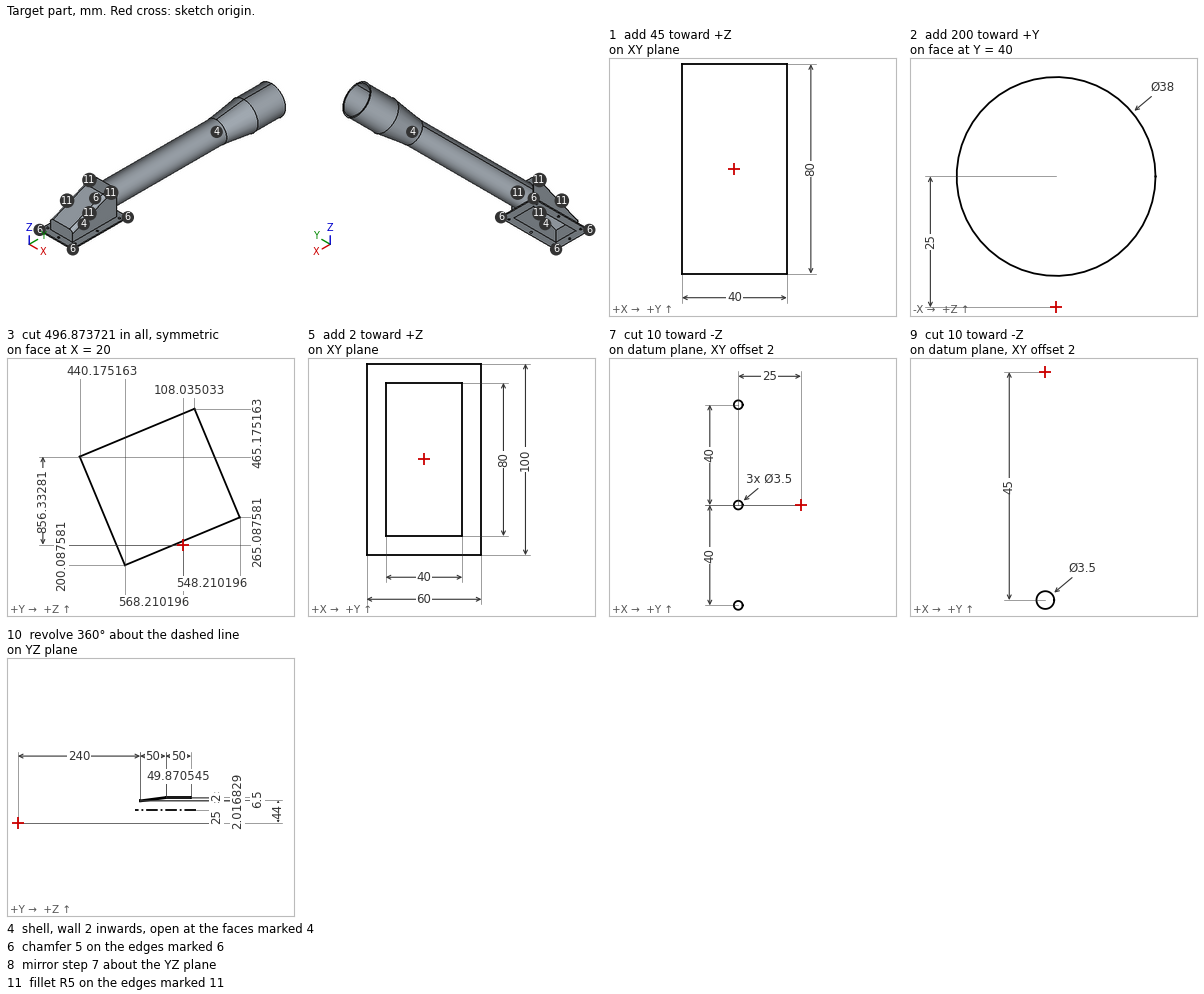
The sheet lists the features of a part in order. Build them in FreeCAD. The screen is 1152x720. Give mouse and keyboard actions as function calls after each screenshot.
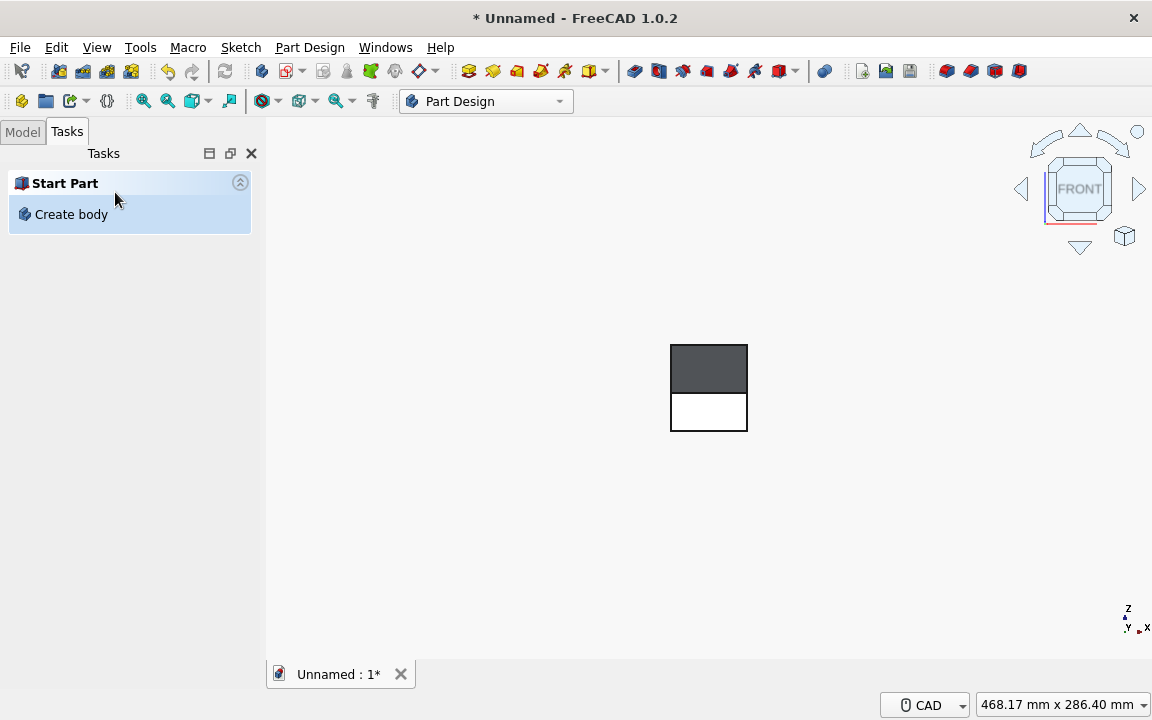
key(3)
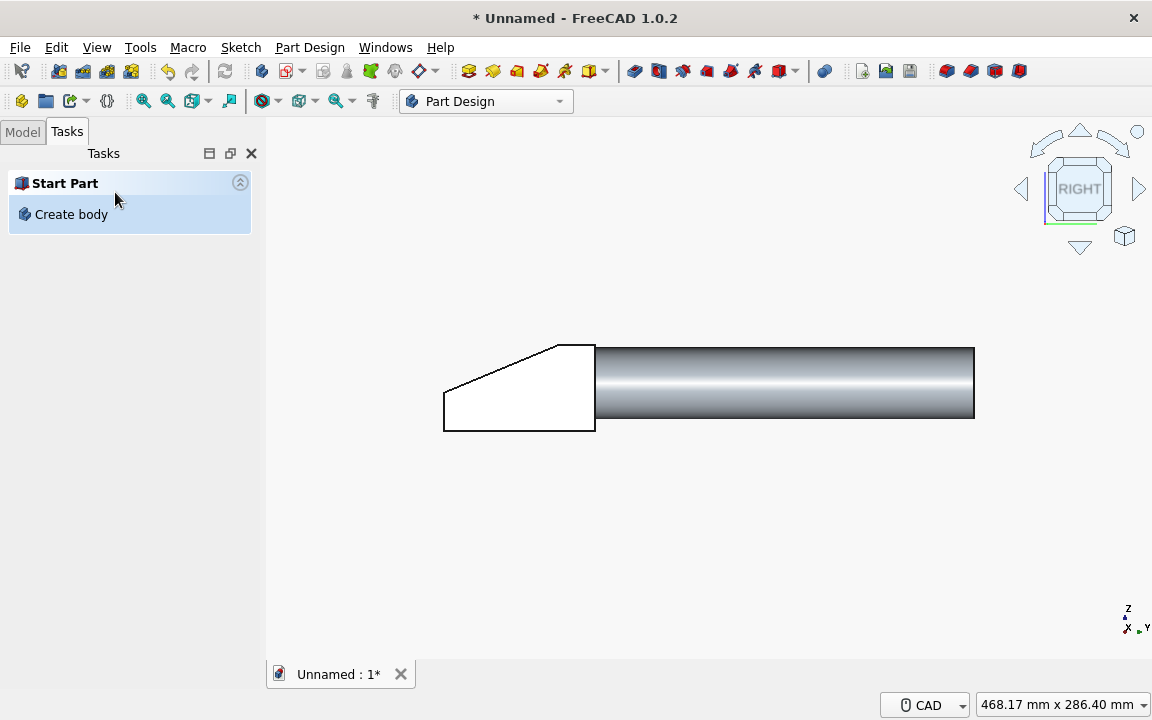
key(5)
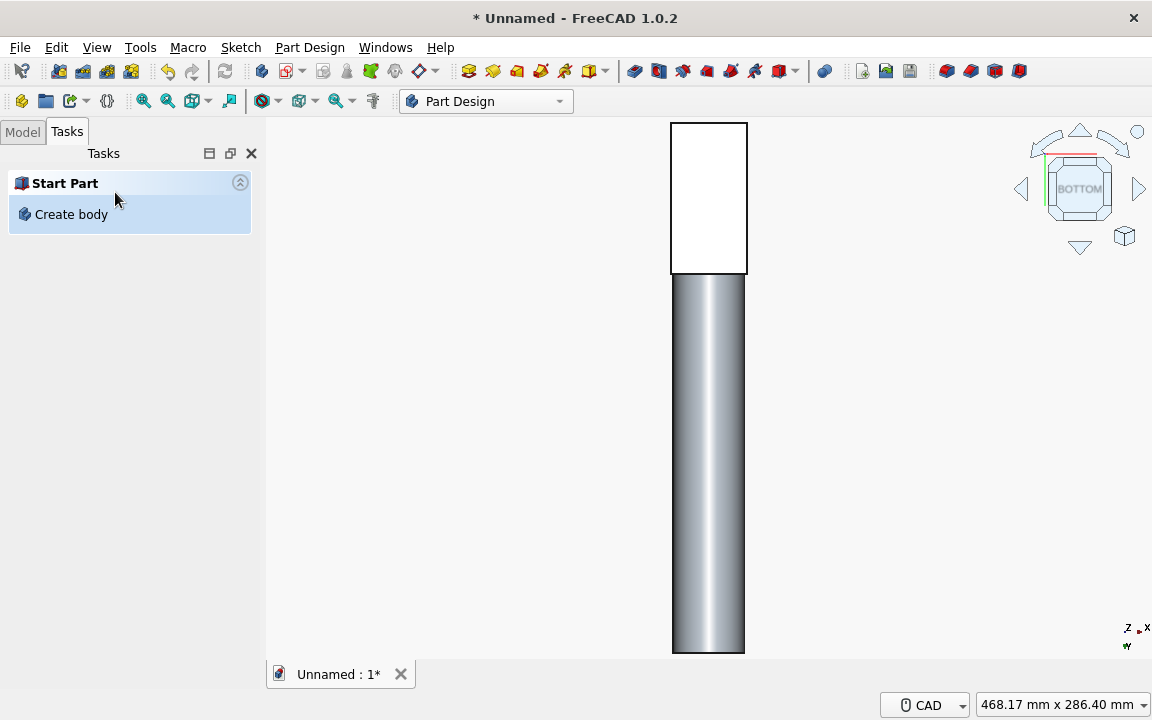
click(709, 219)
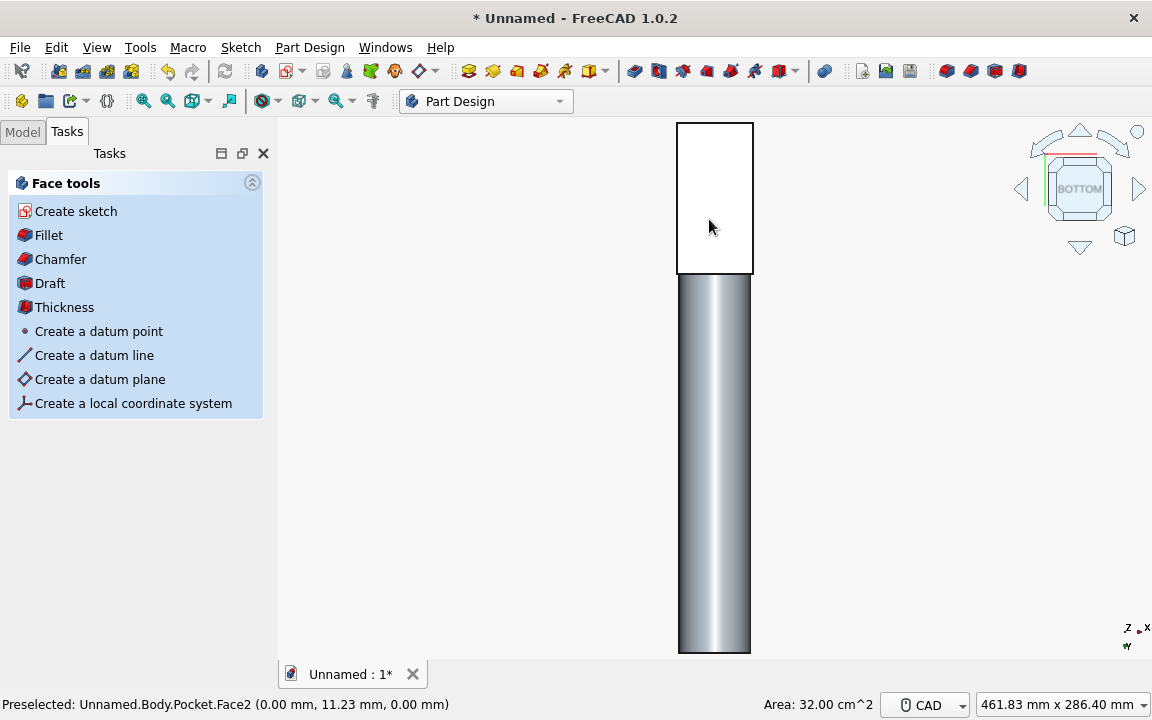
key(4)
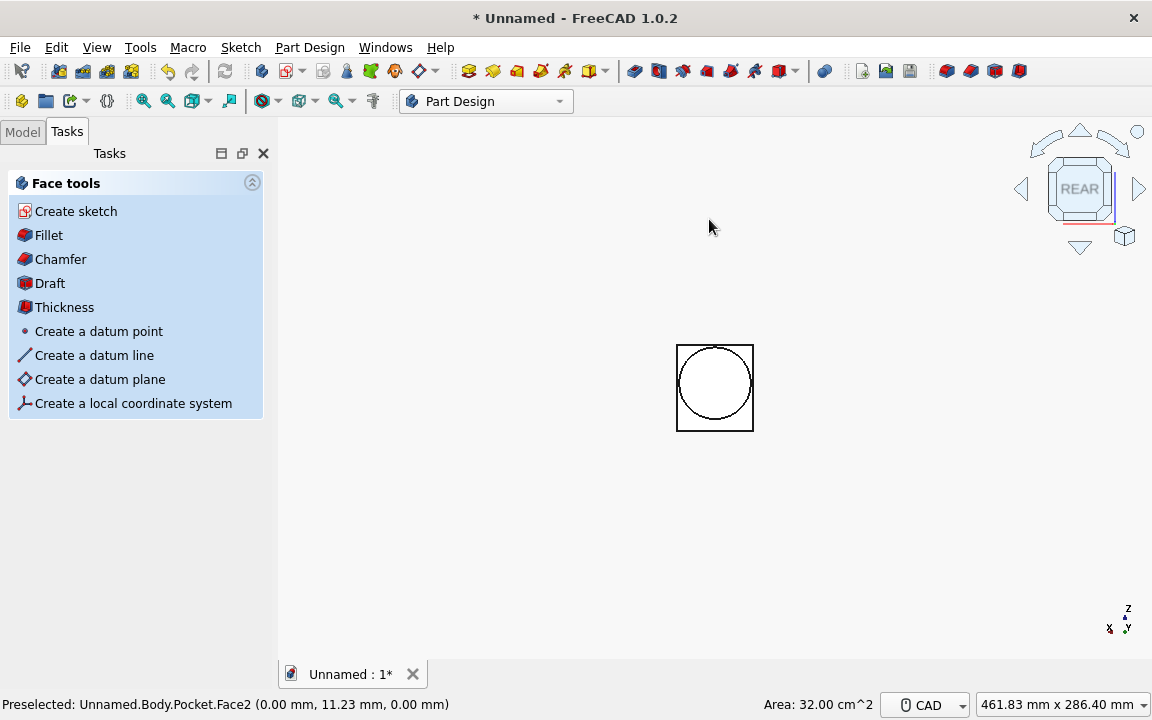
key(v)
key(f)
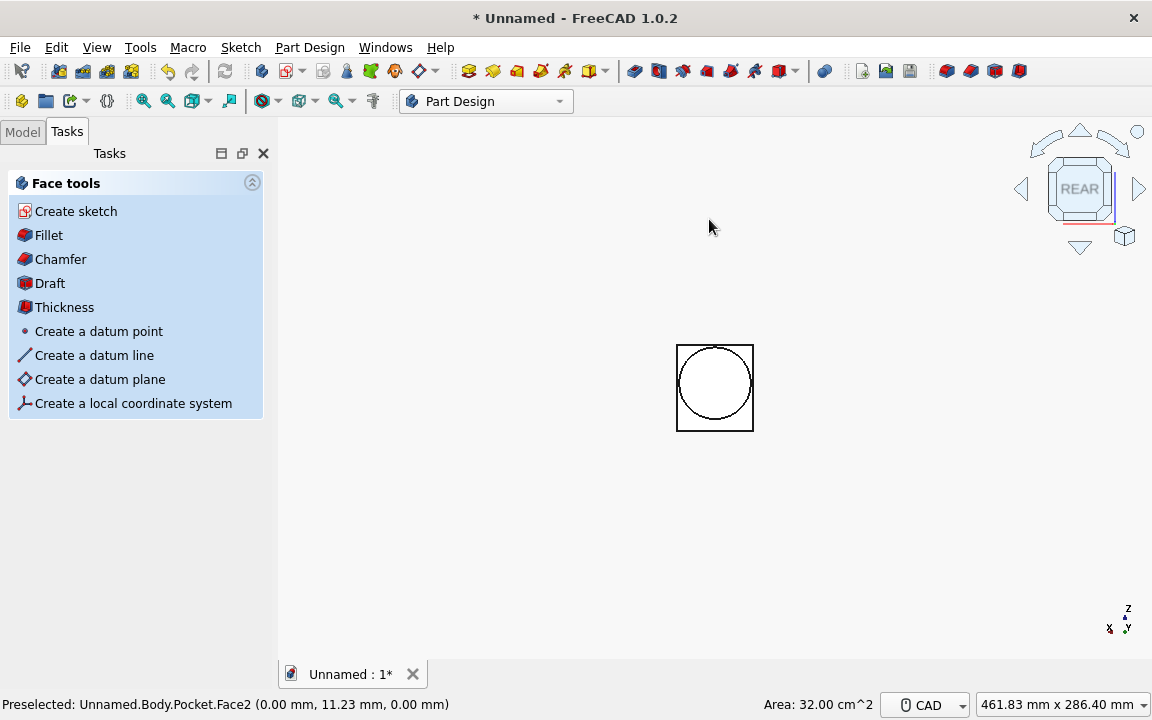
click(715, 382, ctrl)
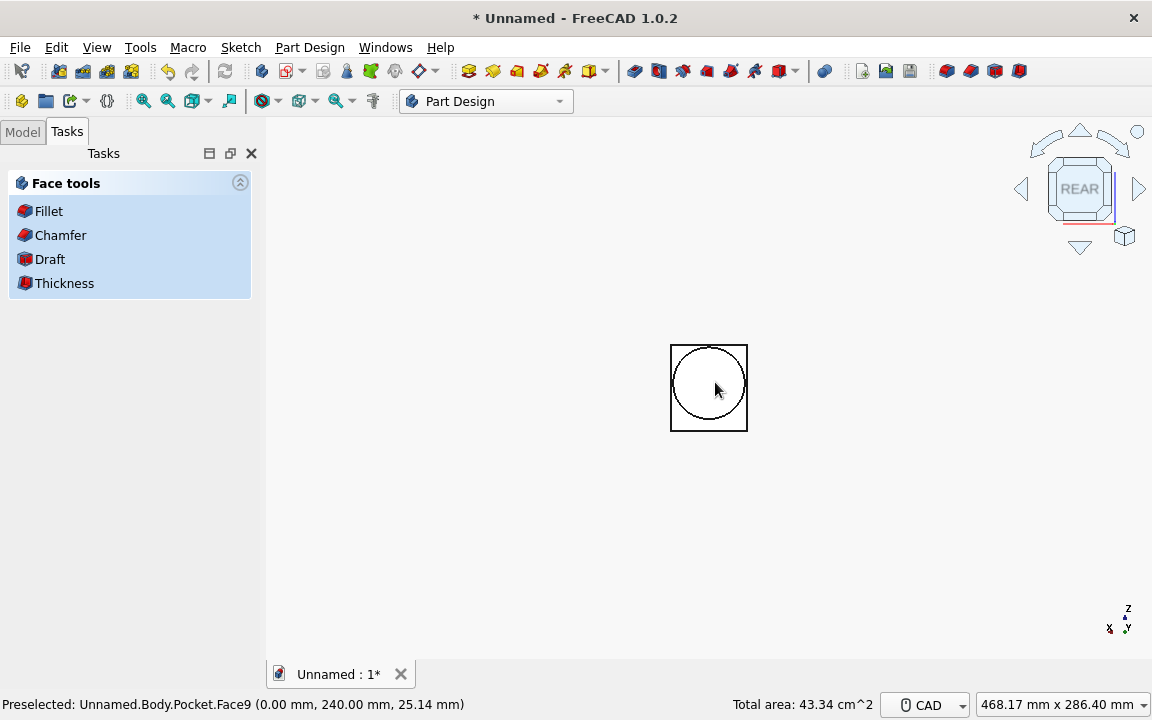
click(1020, 72)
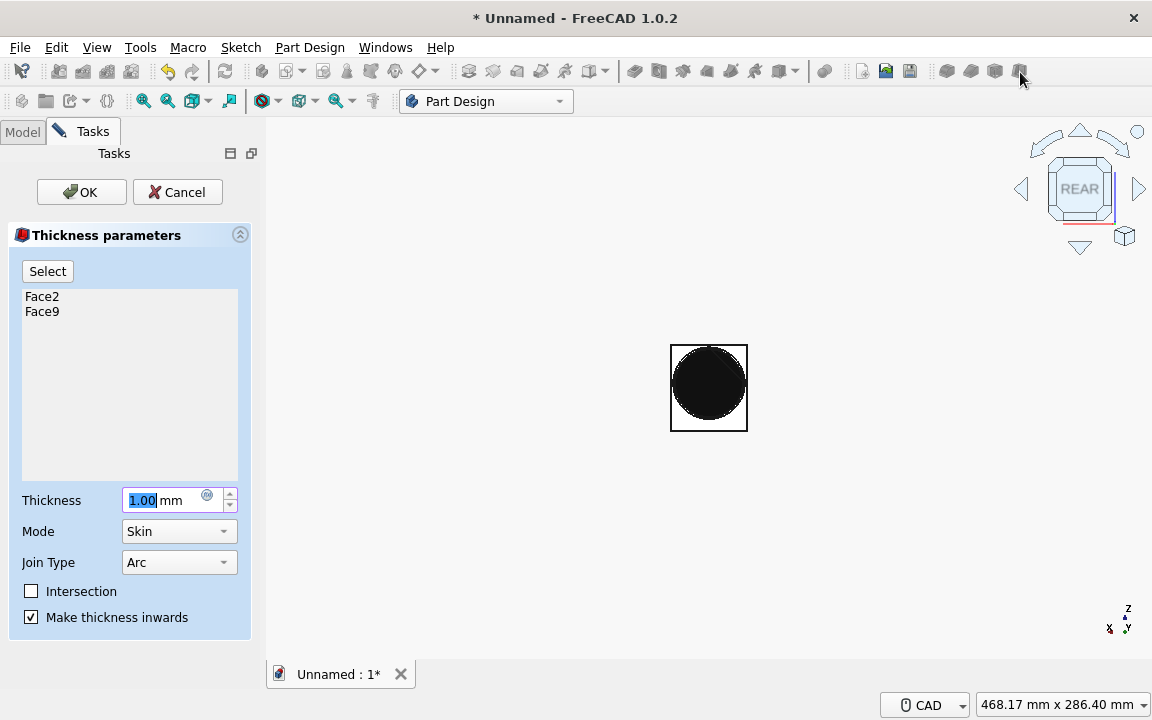
text(2)
key(Tab)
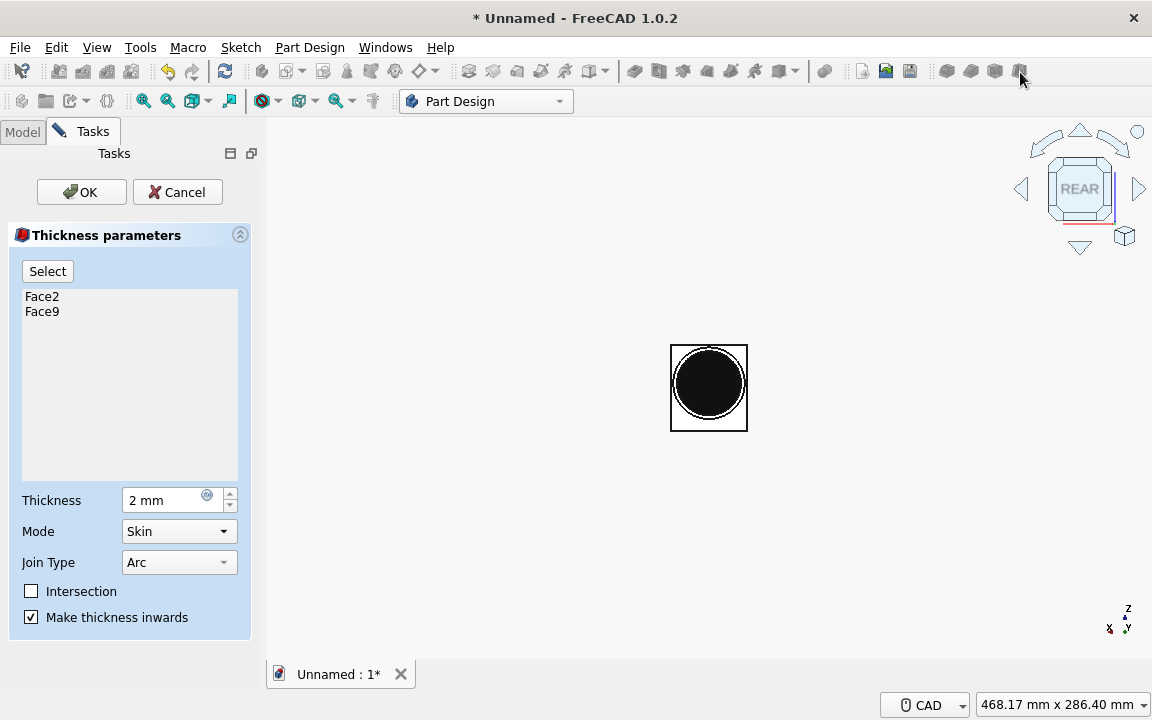
click(180, 562)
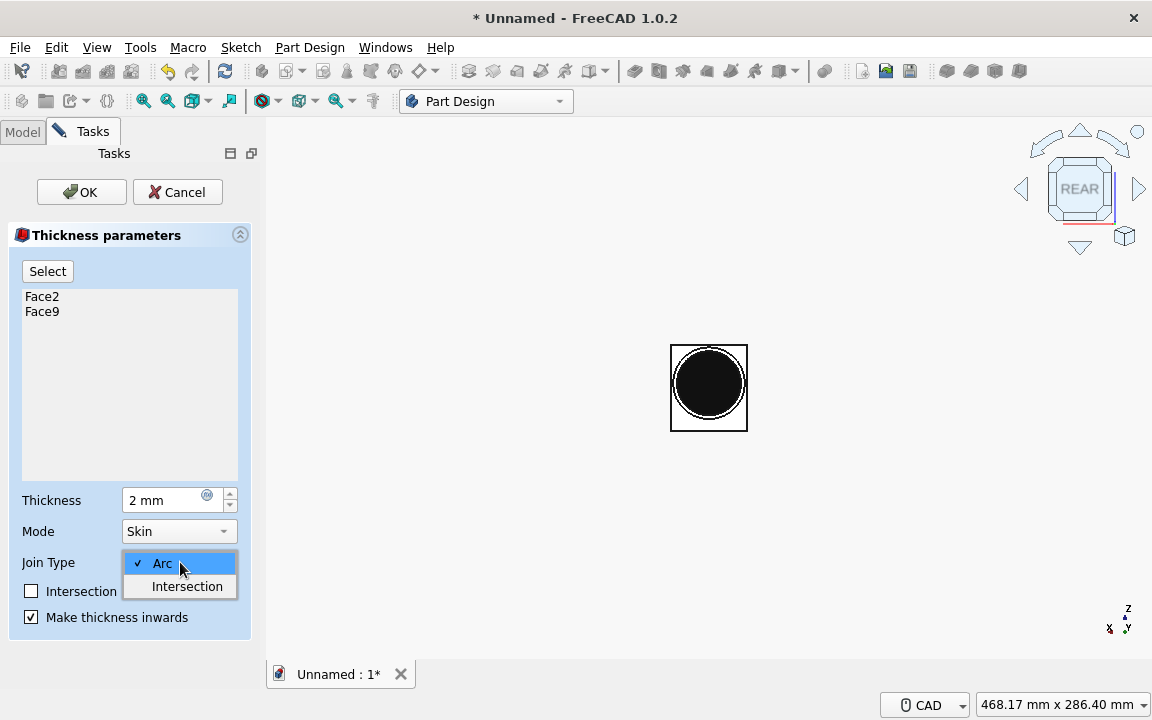
click(179, 586)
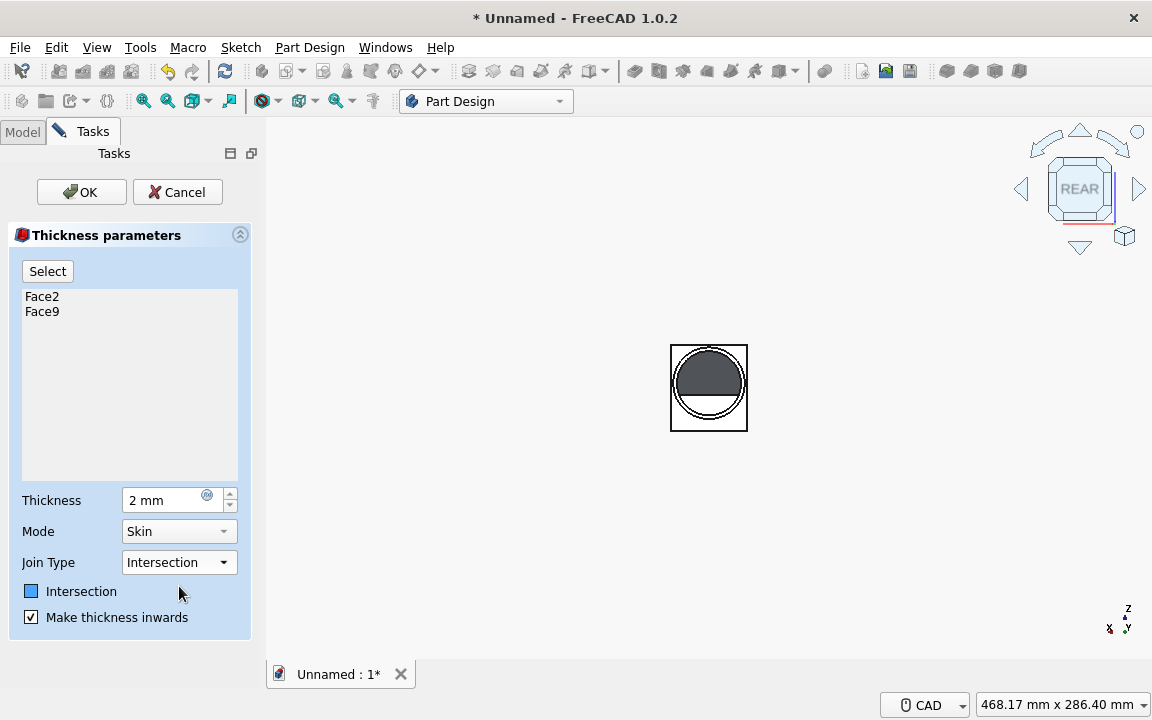
click(82, 192)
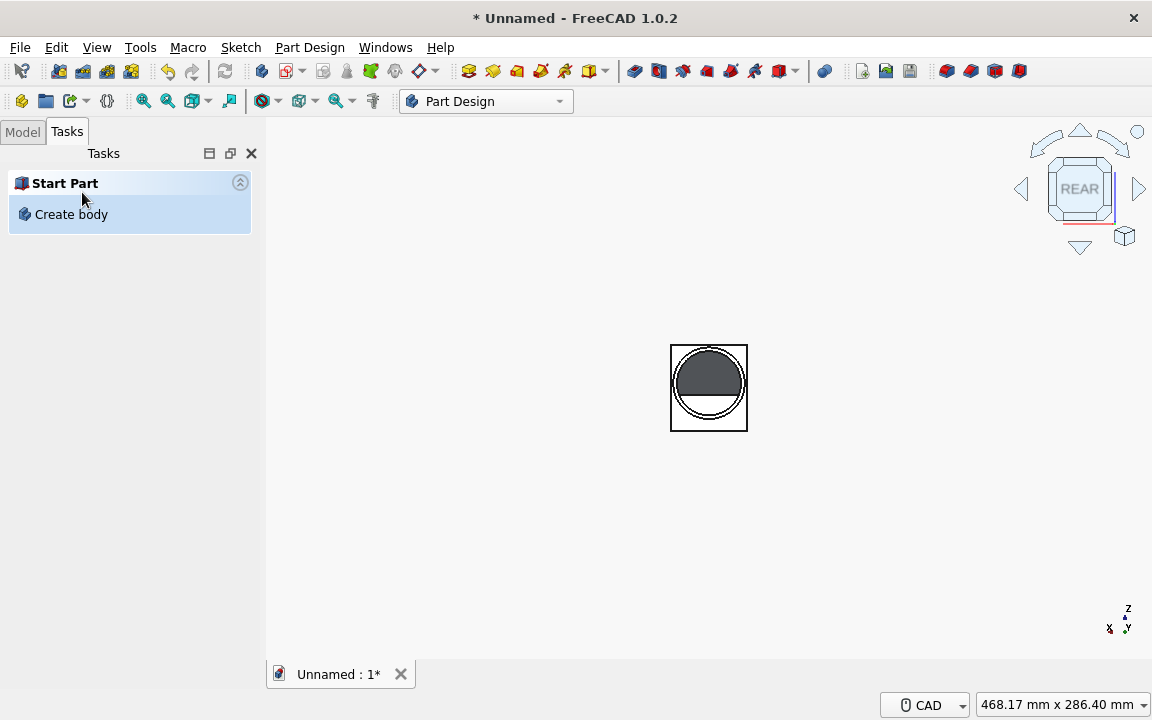
click(144, 102)